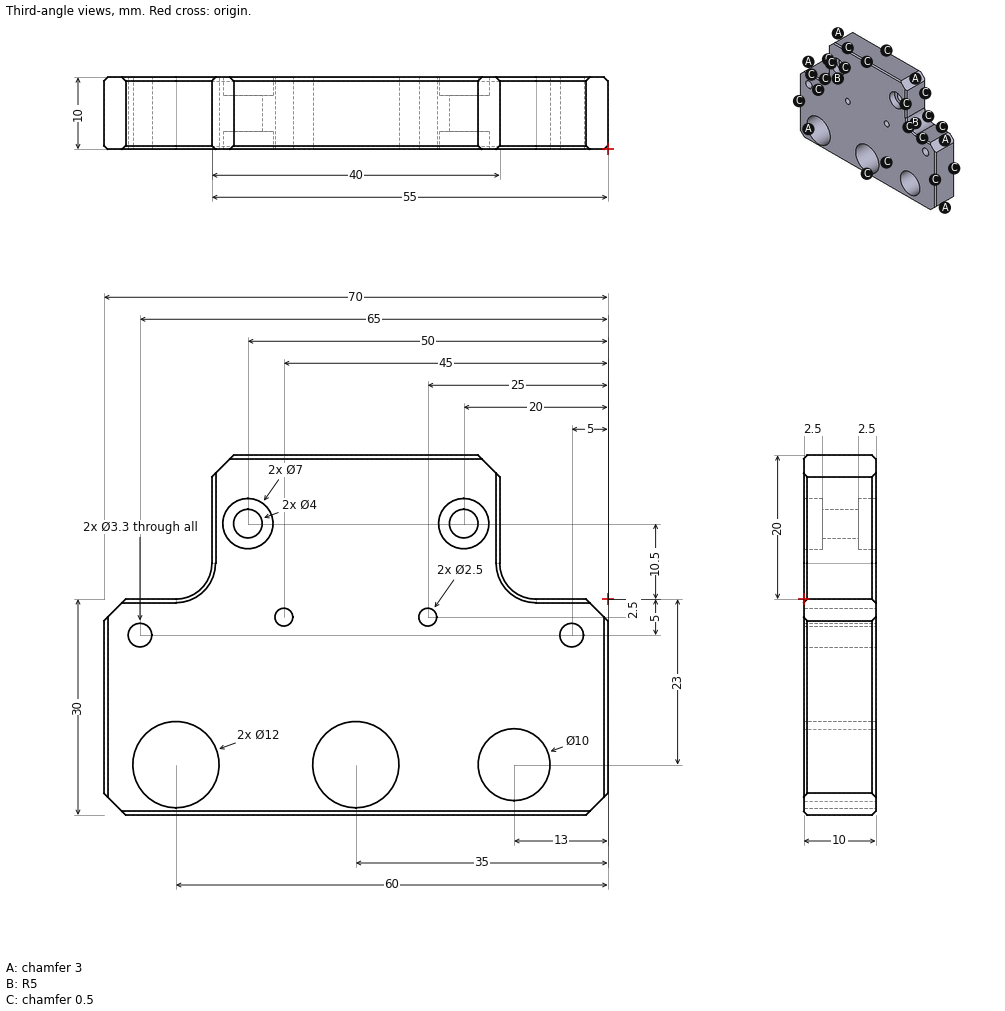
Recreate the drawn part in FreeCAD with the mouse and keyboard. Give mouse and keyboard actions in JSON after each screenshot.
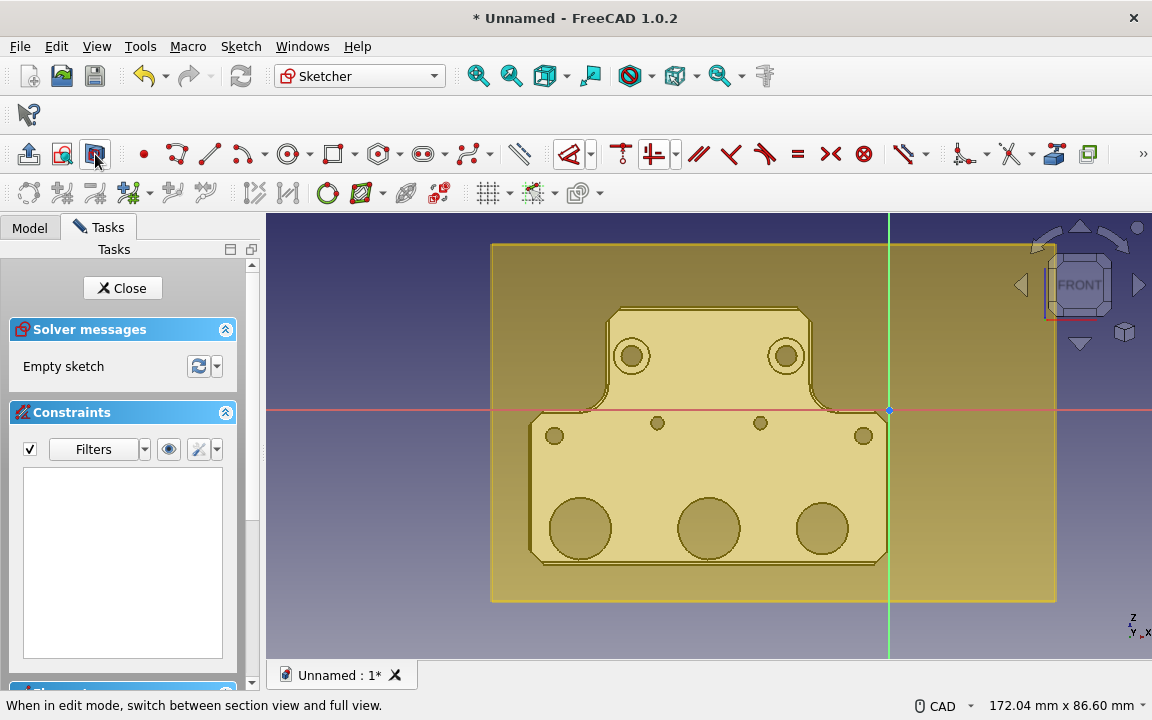
{"action": "scroll", "coordinate": [886, 299], "scroll_direction": "up", "scroll_amount": 3}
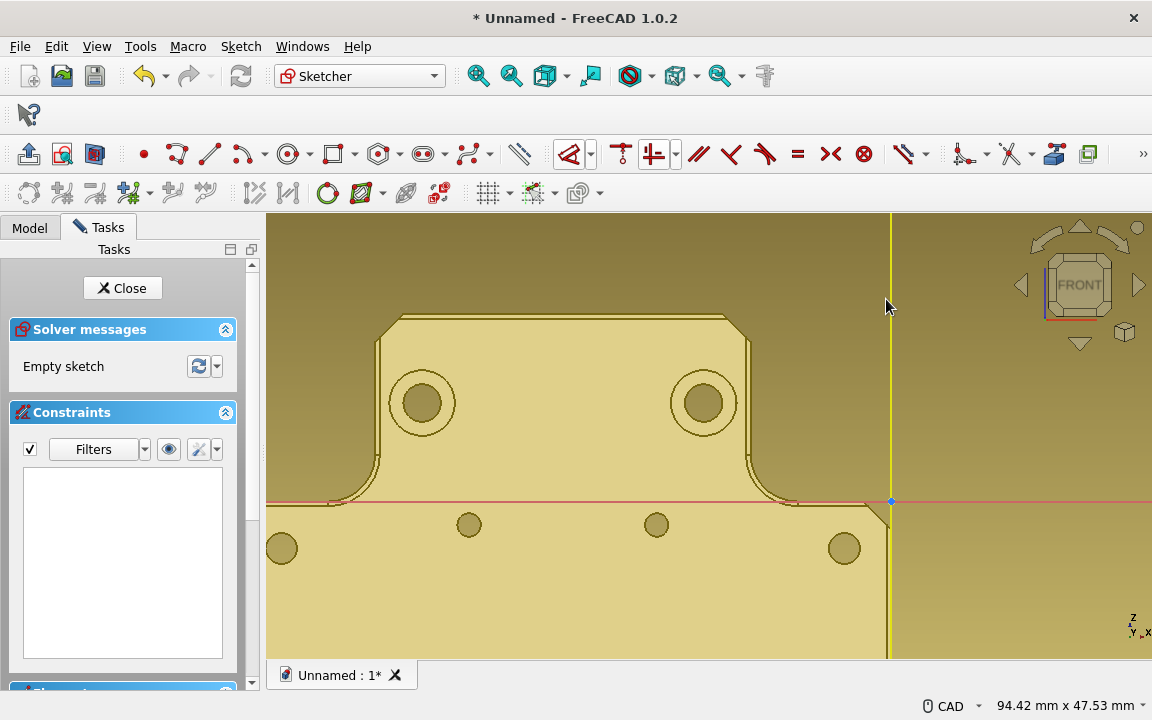
{"action": "left_click", "coordinate": [288, 154]}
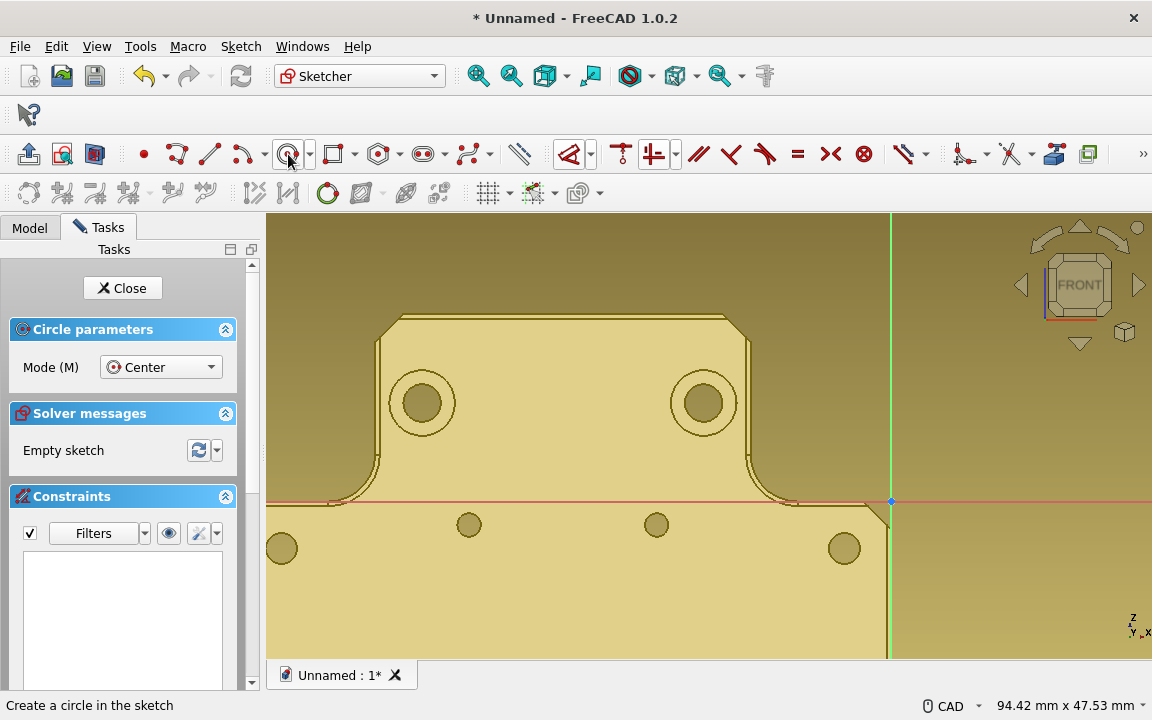
{"action": "left_click", "coordinate": [422, 403]}
{"action": "left_click", "coordinate": [445, 380]}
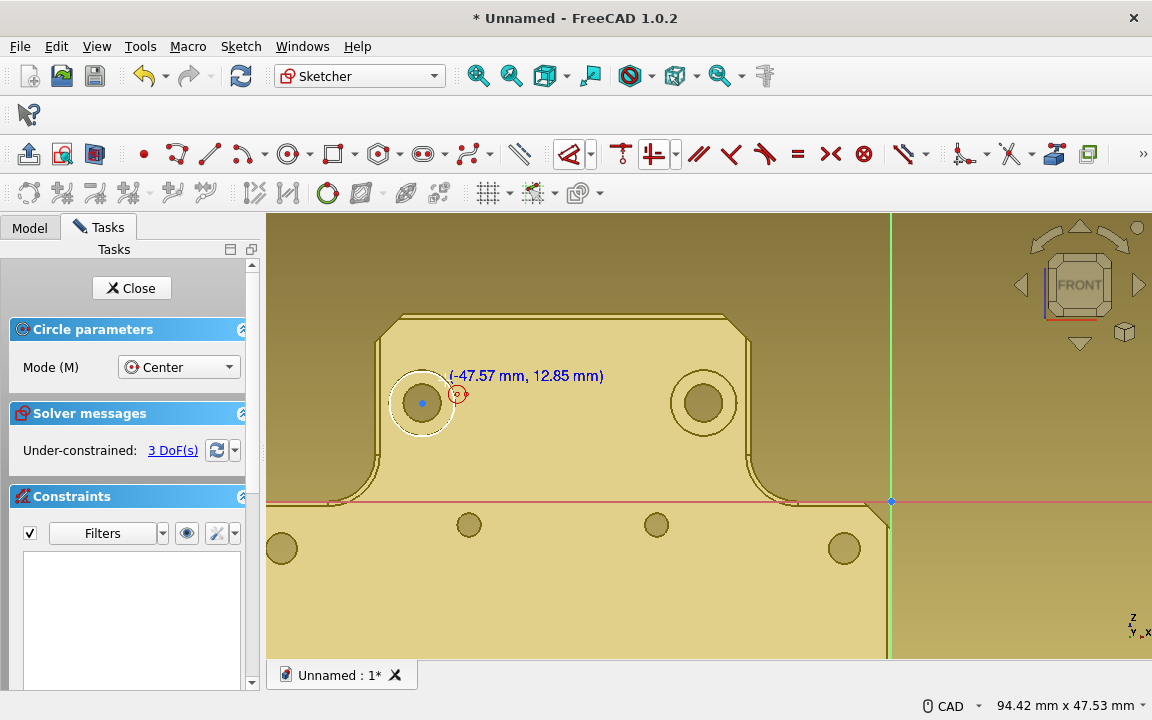
{"action": "left_click", "coordinate": [704, 403]}
{"action": "left_click", "coordinate": [727, 380]}
{"action": "key", "text": "Escape"}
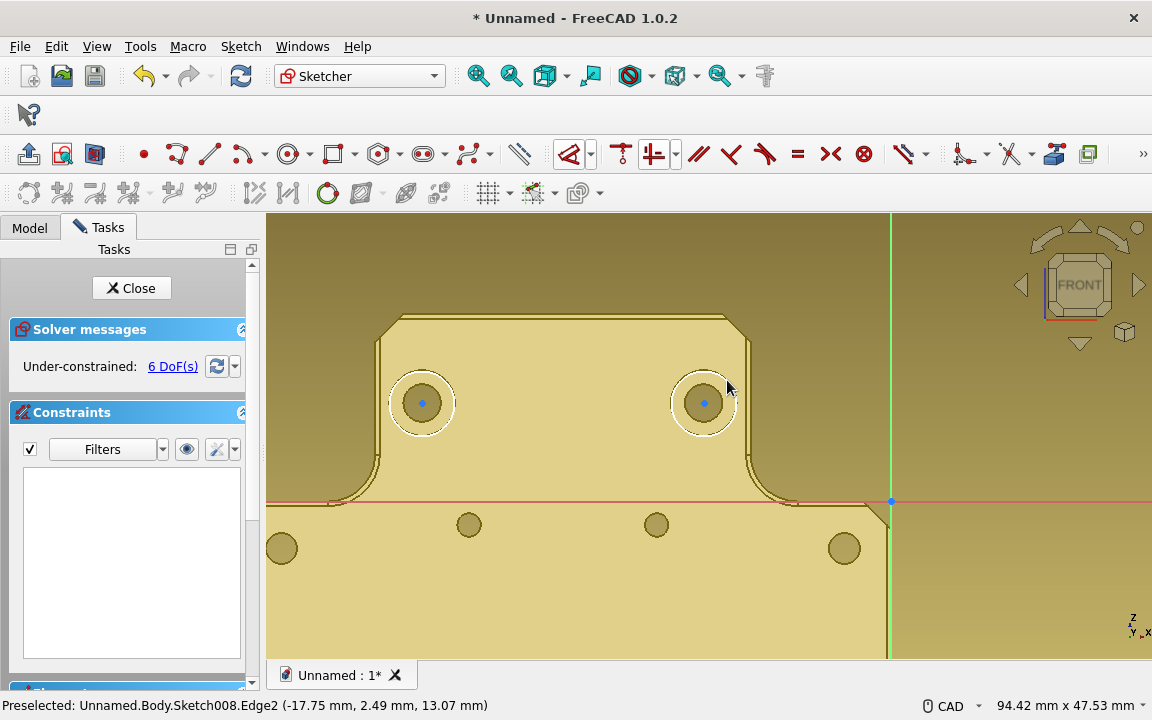
{"action": "left_click", "coordinate": [445, 381]}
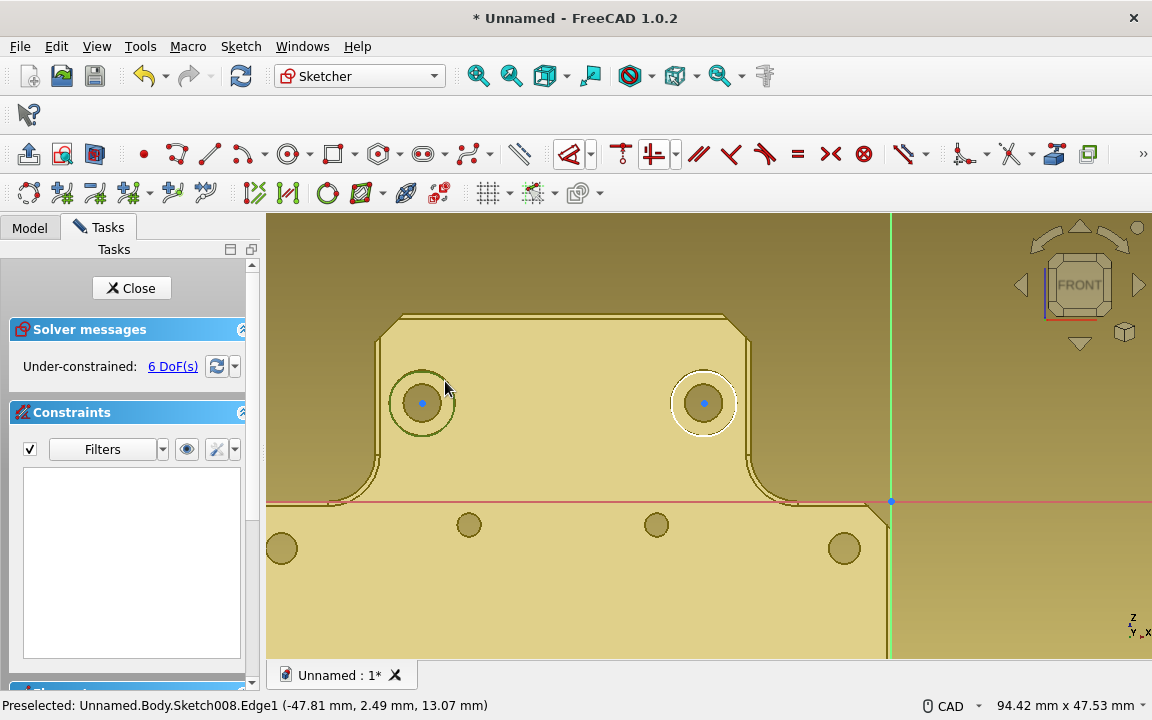
{"action": "left_click", "coordinate": [727, 381]}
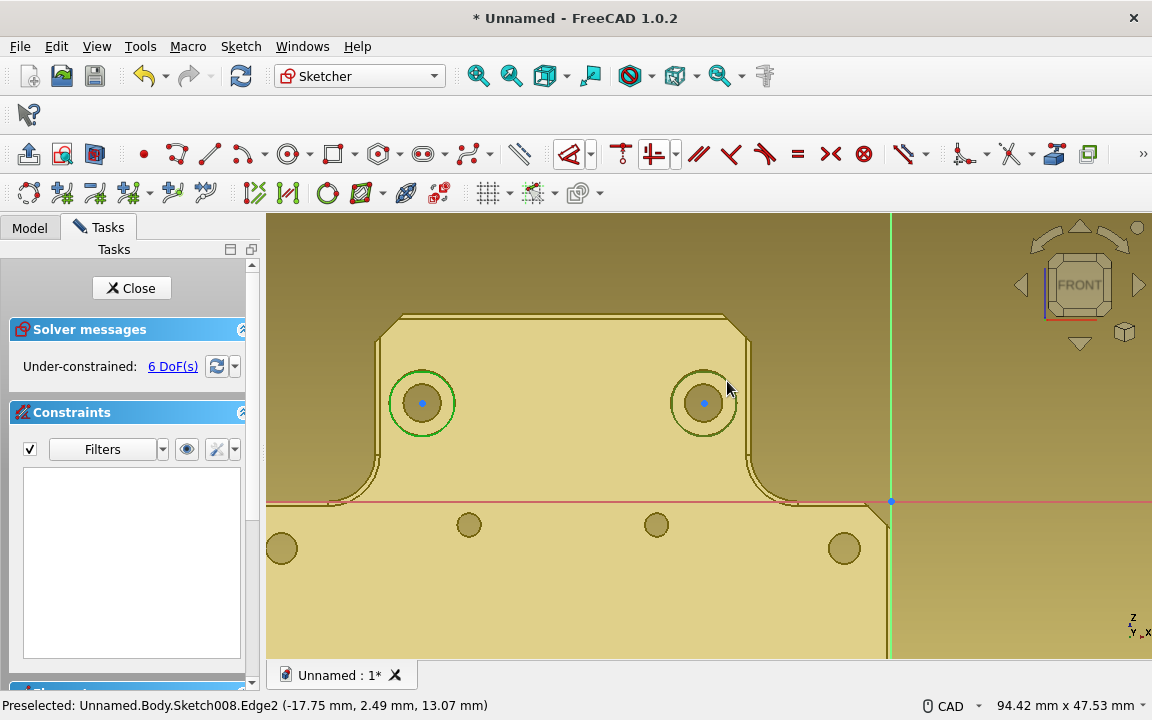
{"action": "left_click", "coordinate": [798, 154]}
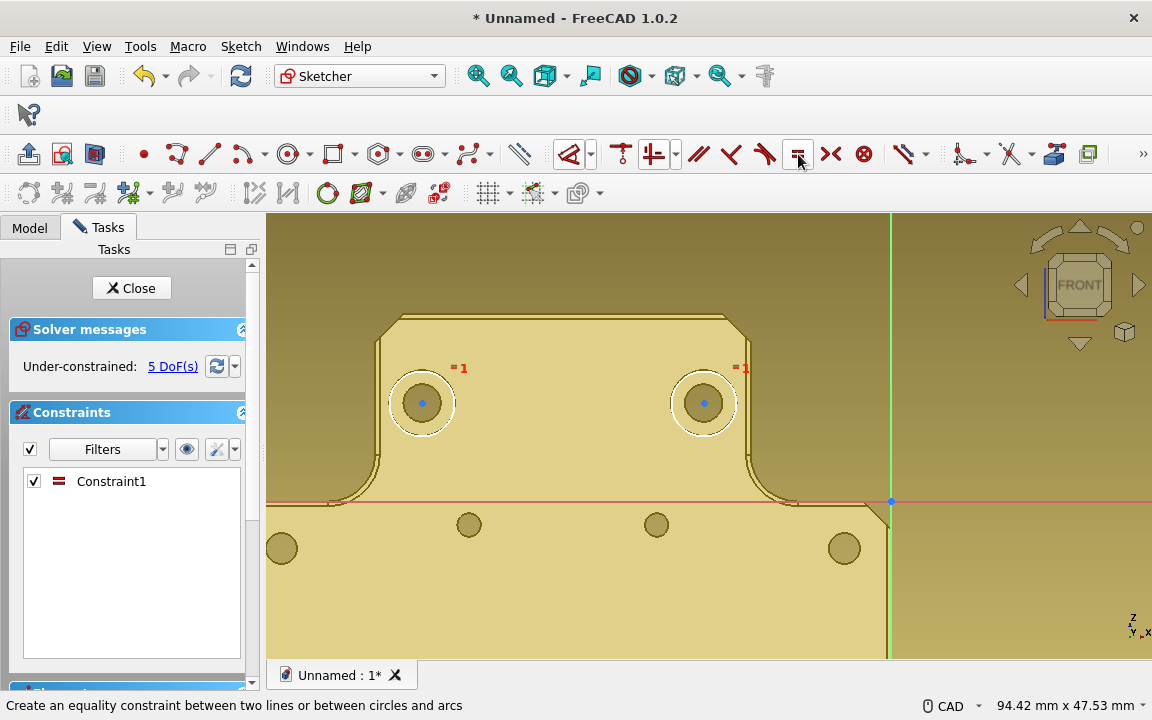
{"action": "left_click", "coordinate": [422, 404]}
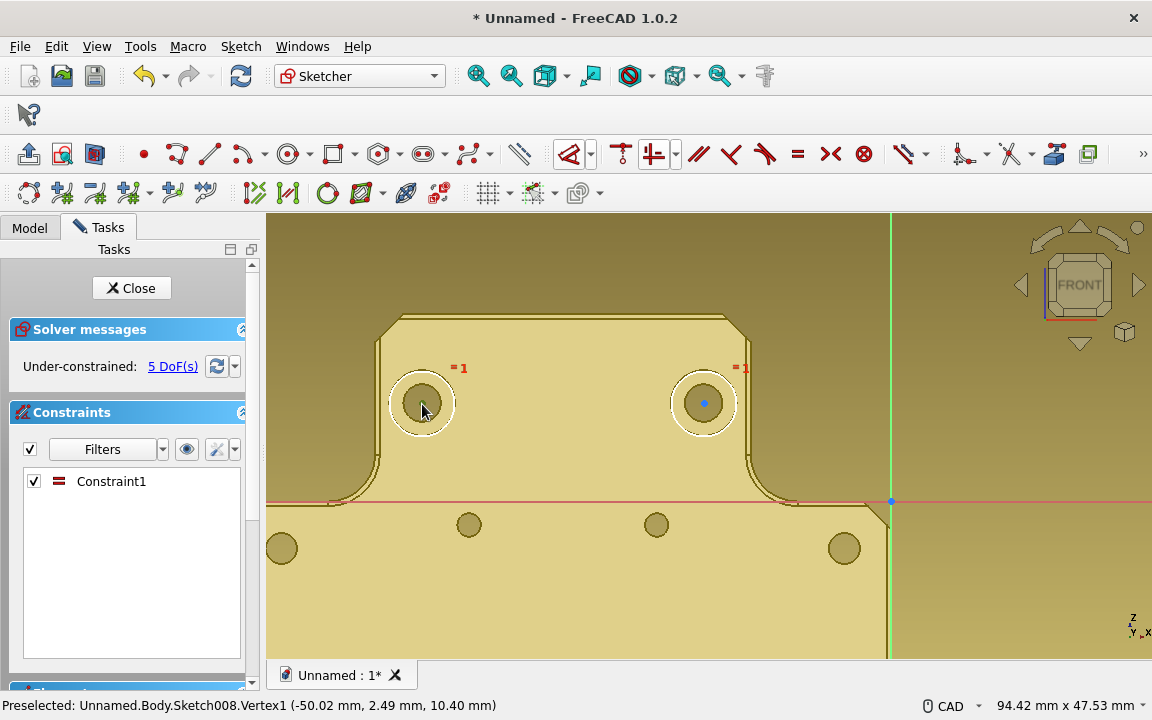
{"action": "left_click", "coordinate": [704, 404]}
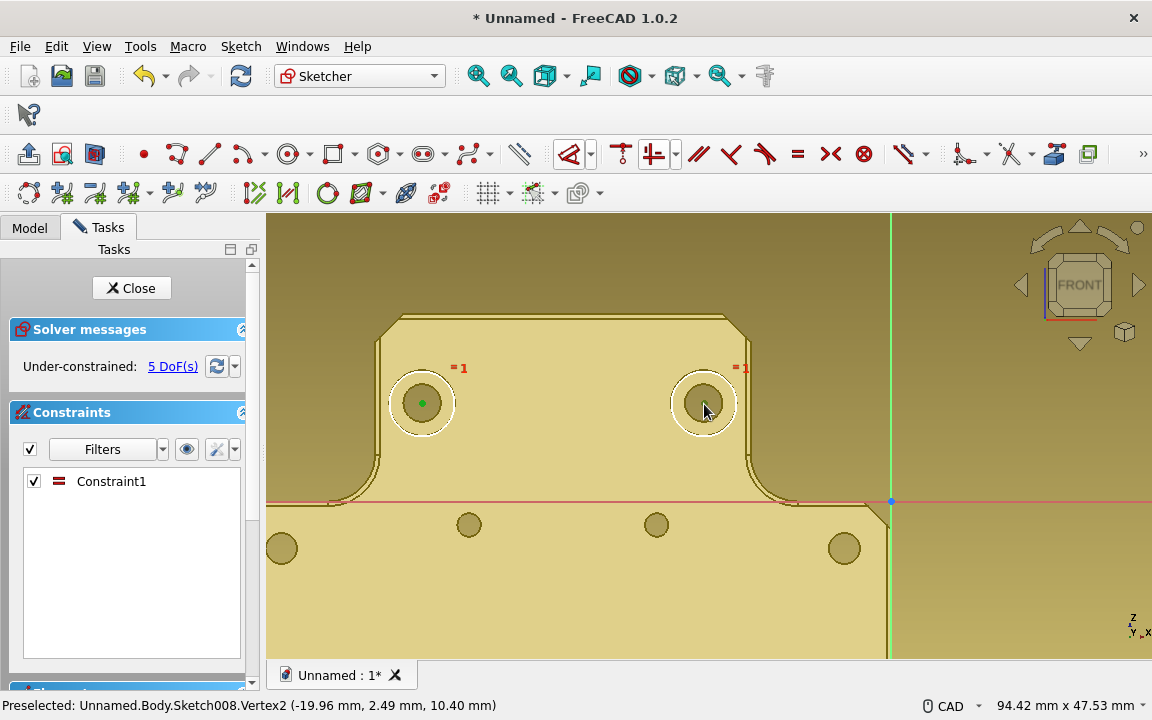
{"action": "key", "text": "h"}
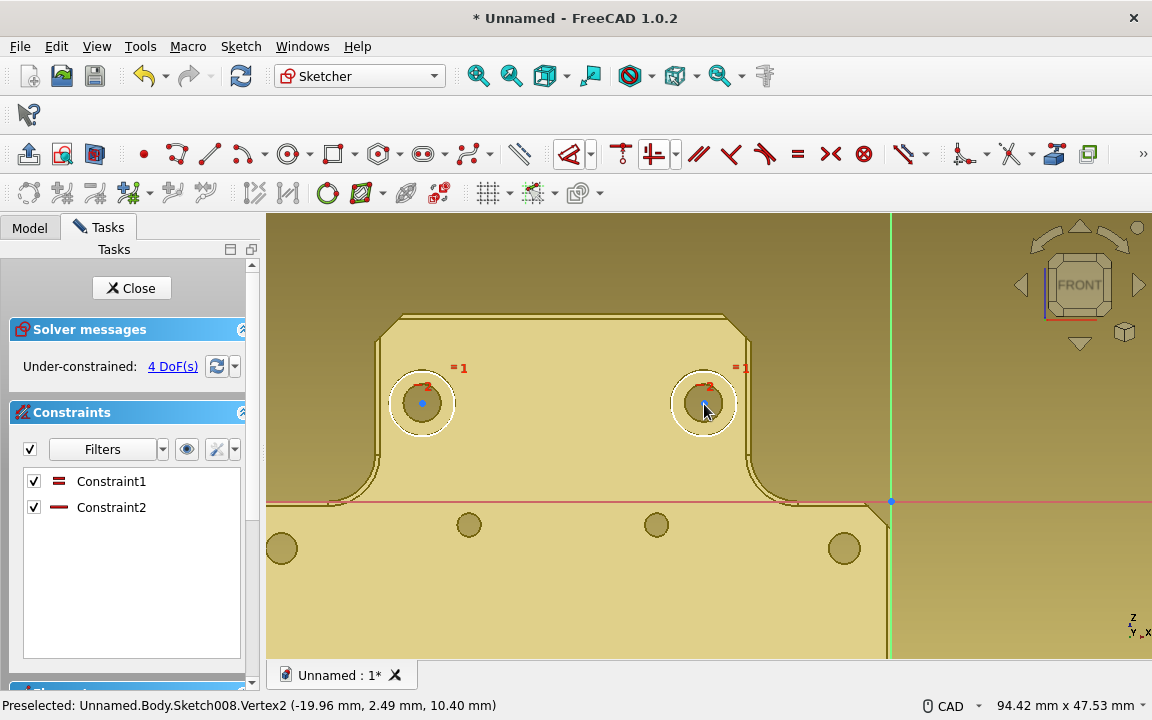
{"action": "left_click", "coordinate": [445, 381]}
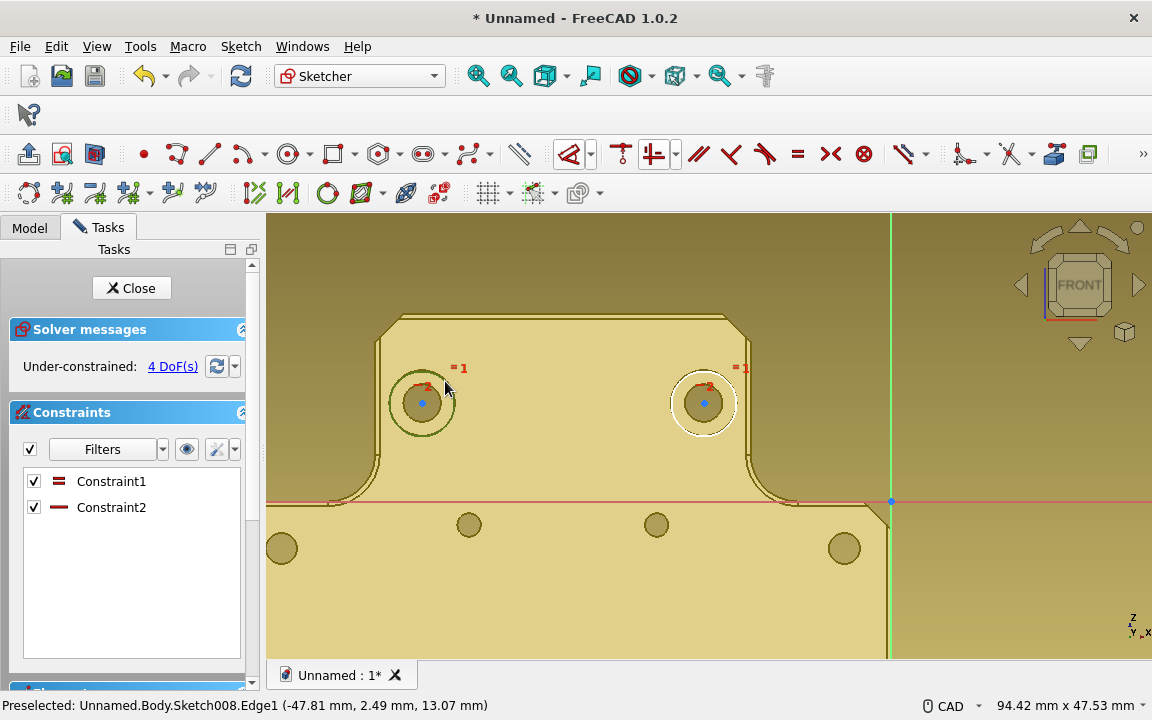
{"action": "left_click", "coordinate": [590, 154]}